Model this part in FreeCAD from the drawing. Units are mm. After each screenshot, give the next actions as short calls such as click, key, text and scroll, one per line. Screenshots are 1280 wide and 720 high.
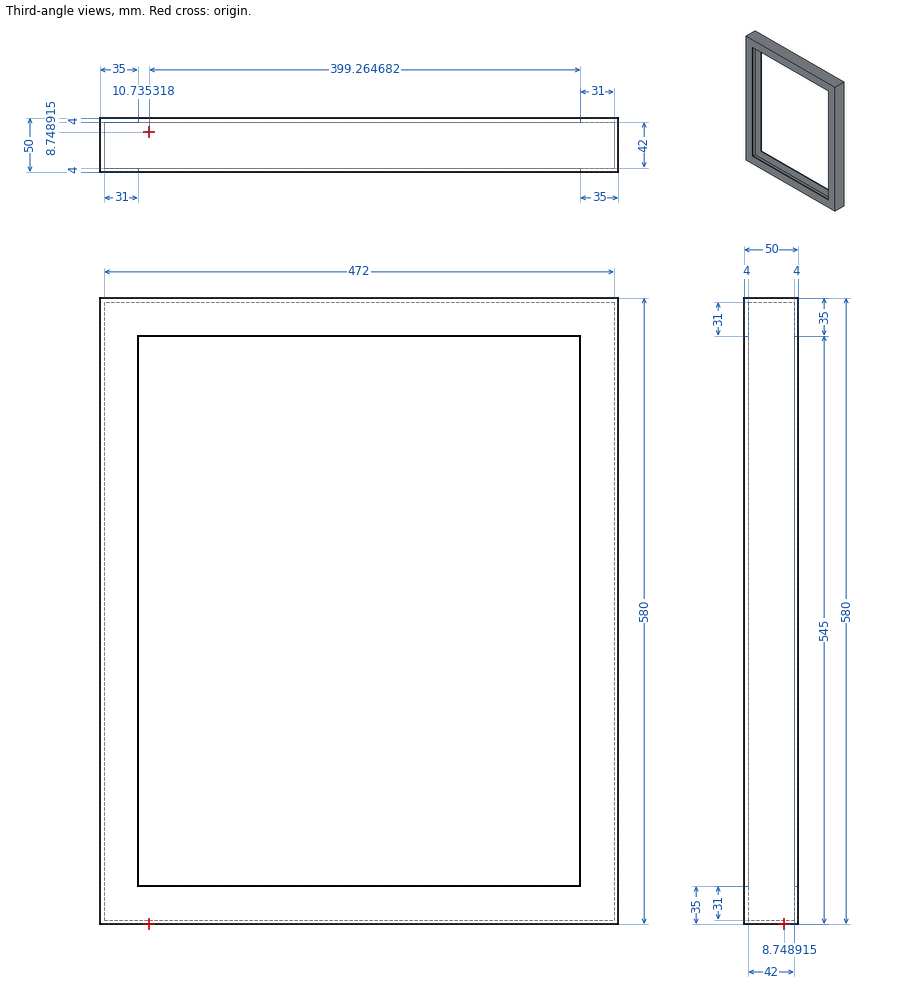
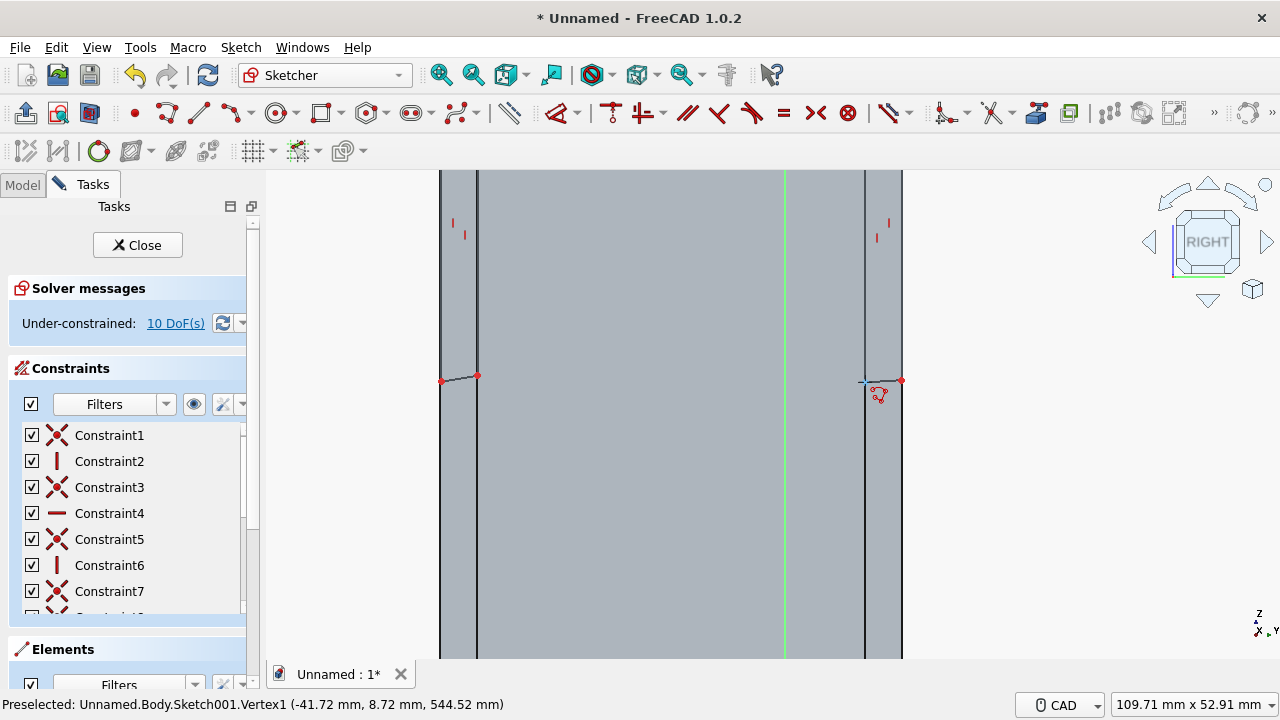
scroll(707, 264, down, 14)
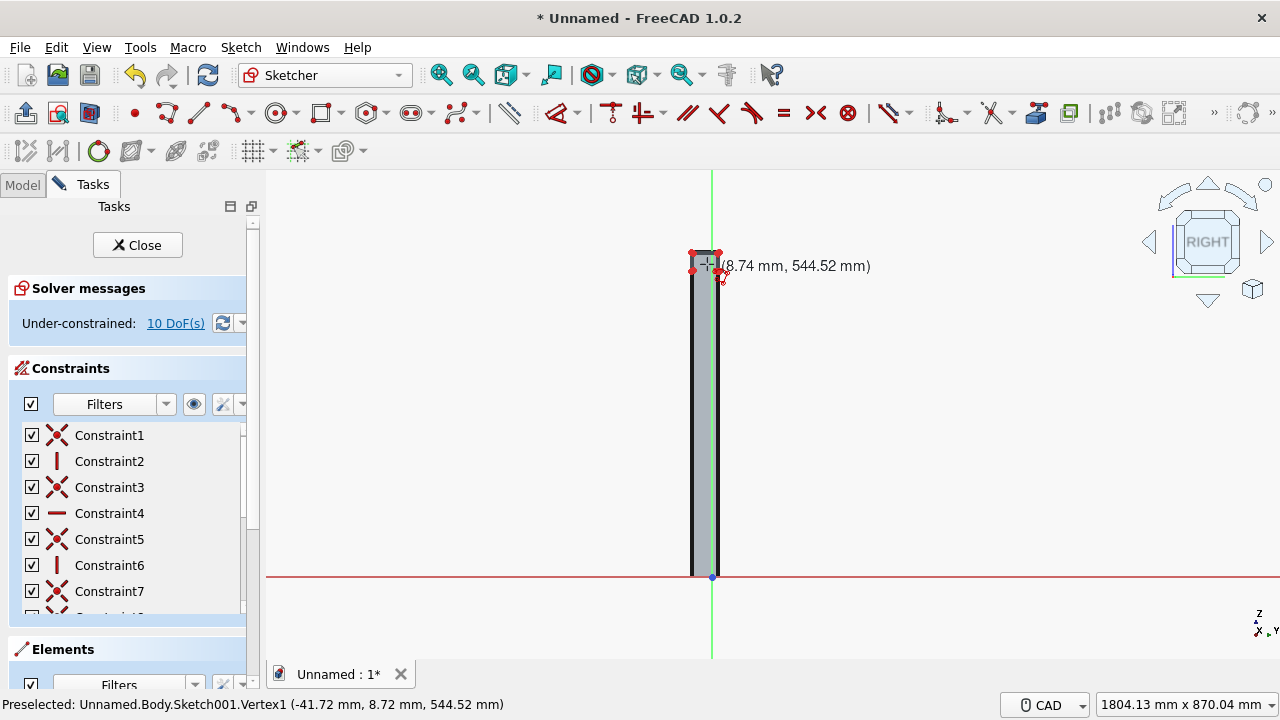
scroll(717, 575, up, 10)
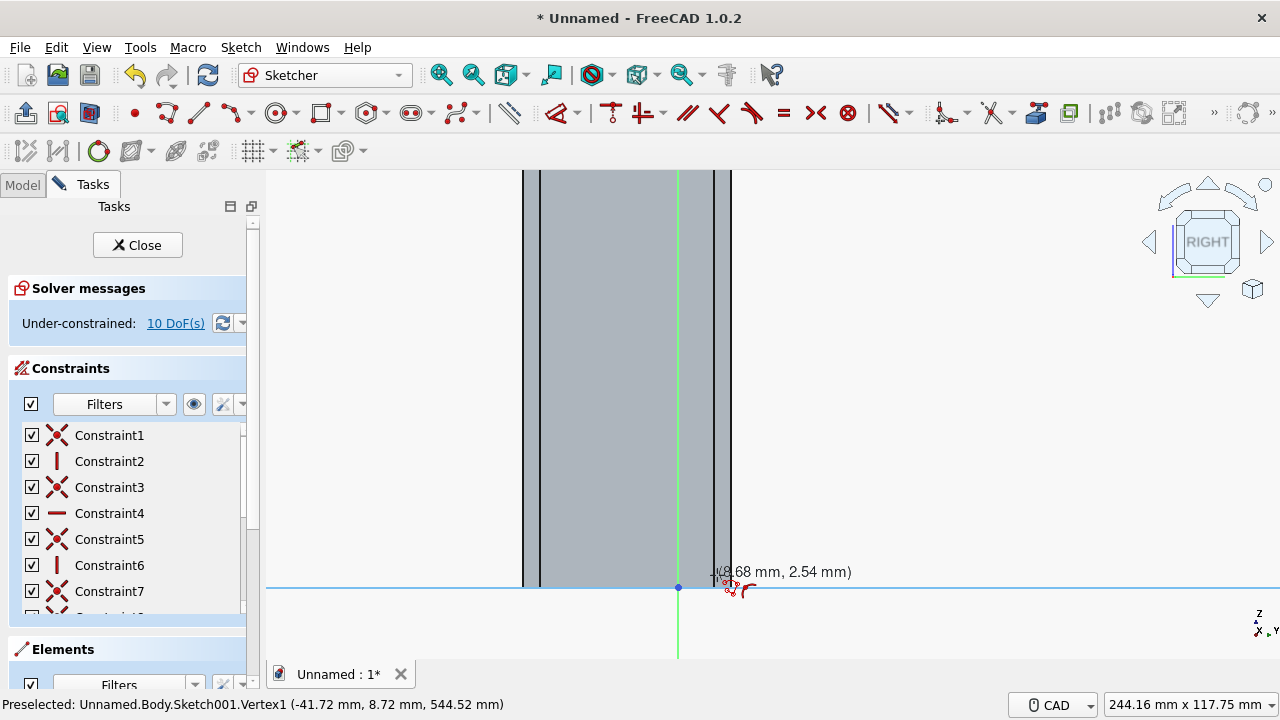
click(714, 571)
click(540, 571)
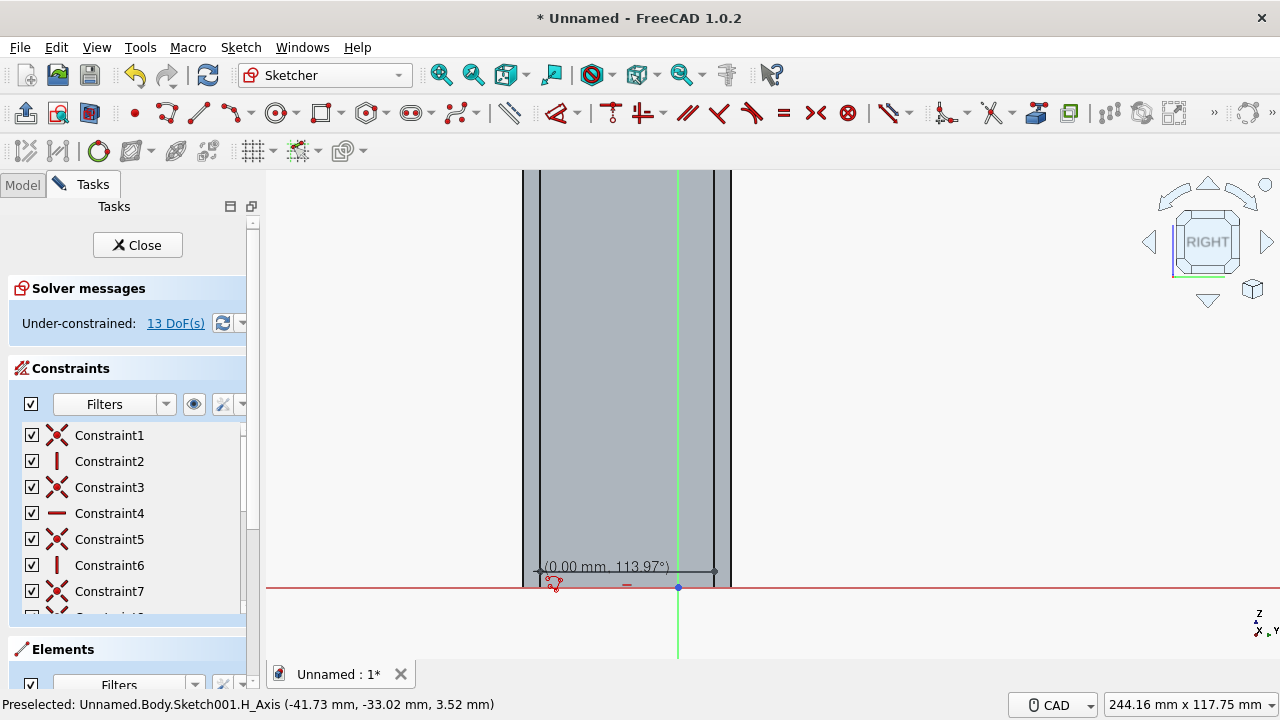
scroll(717, 576, down, 10)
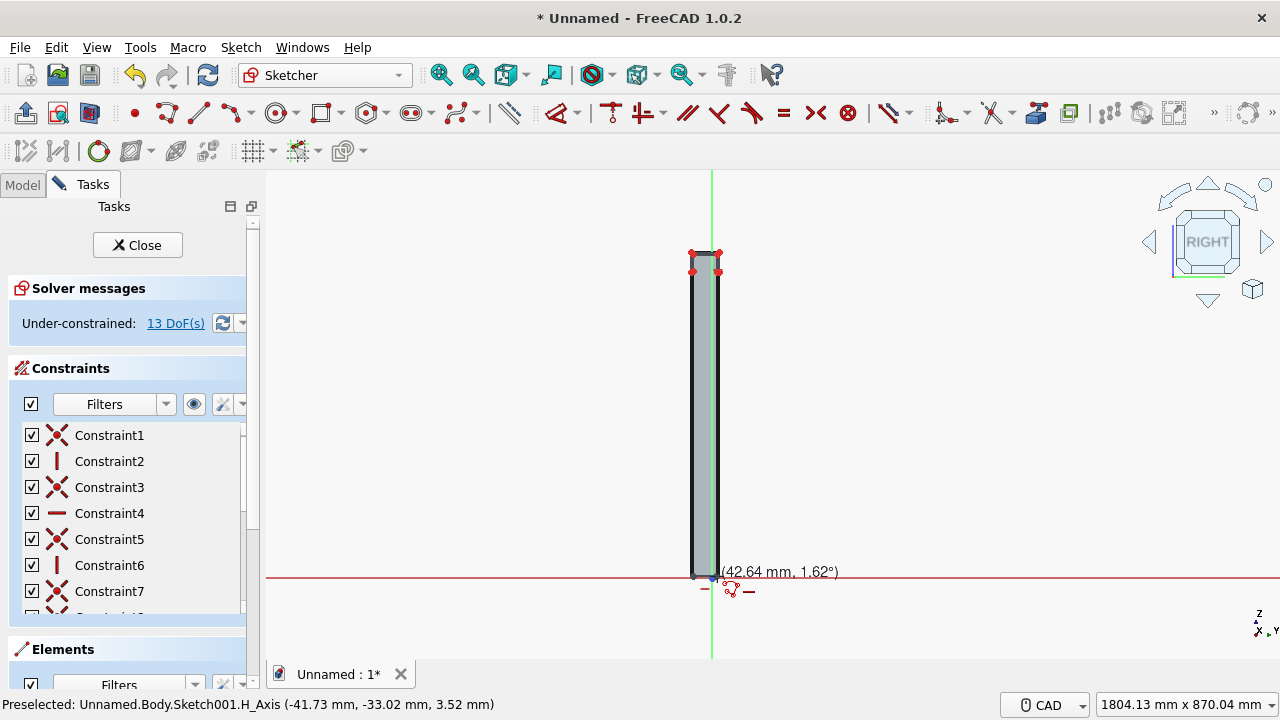
click(693, 559)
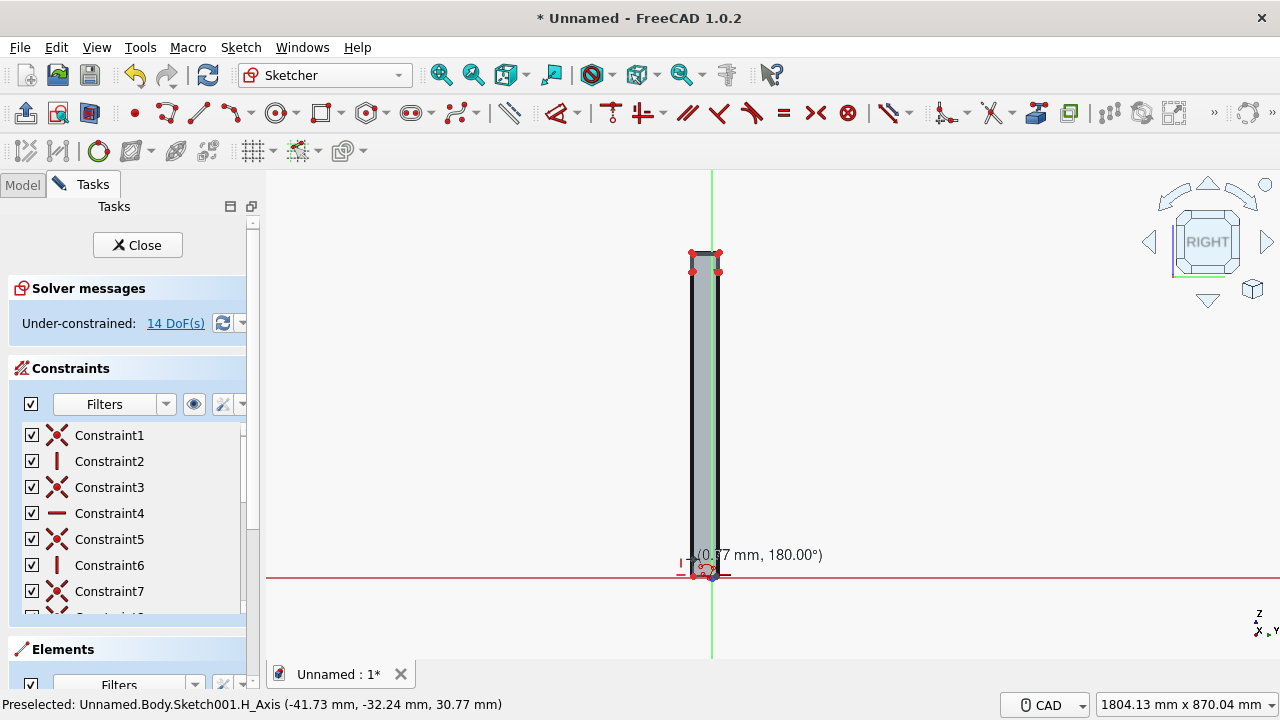
scroll(691, 559, up, 10)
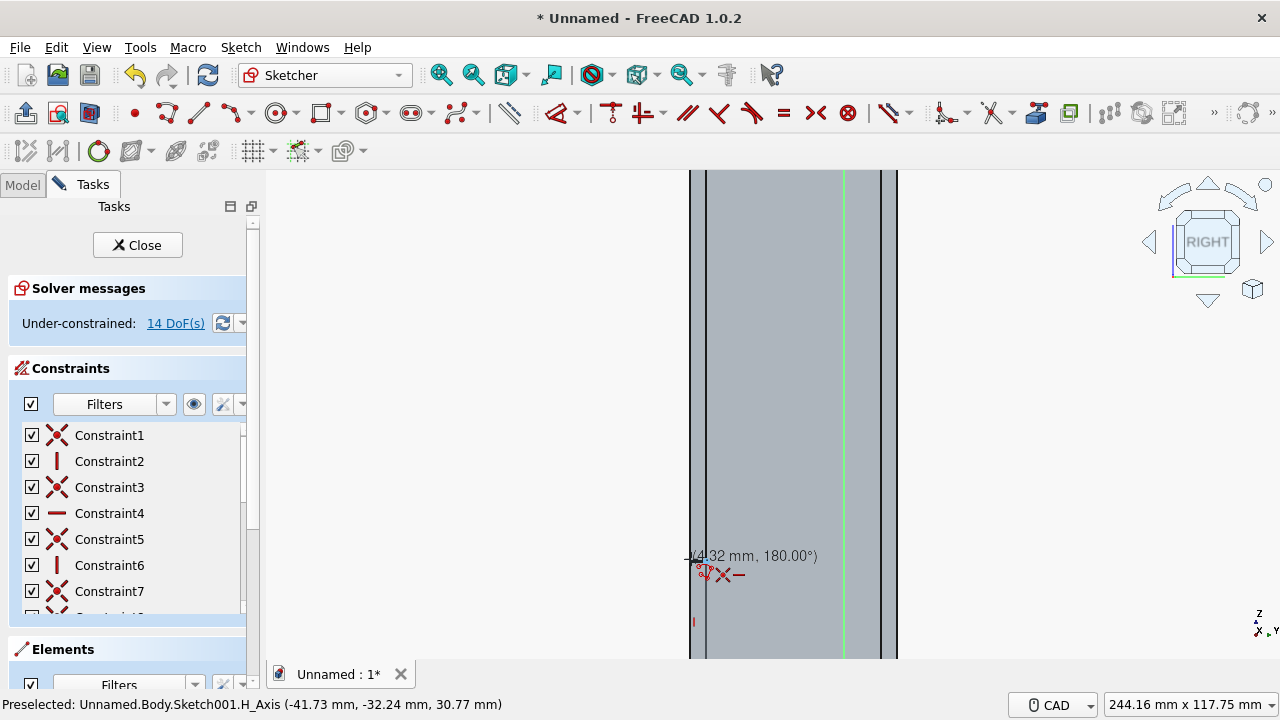
click(690, 554)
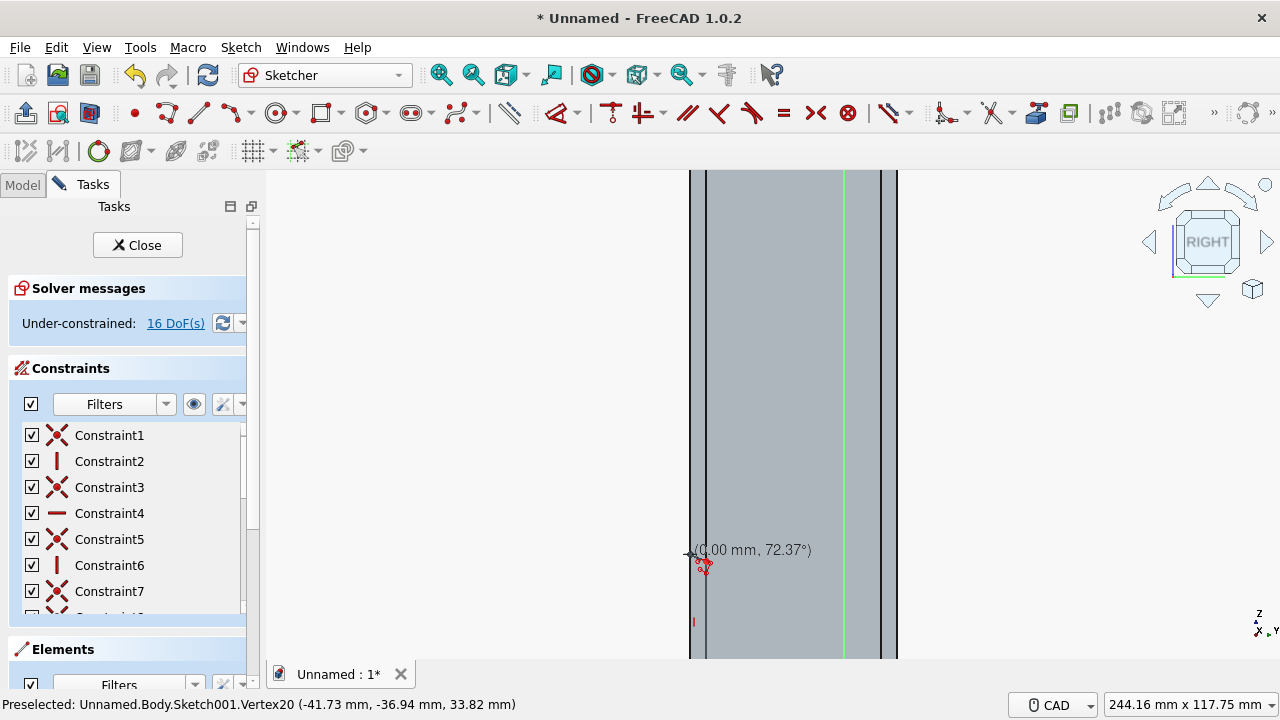
scroll(691, 559, down, 10)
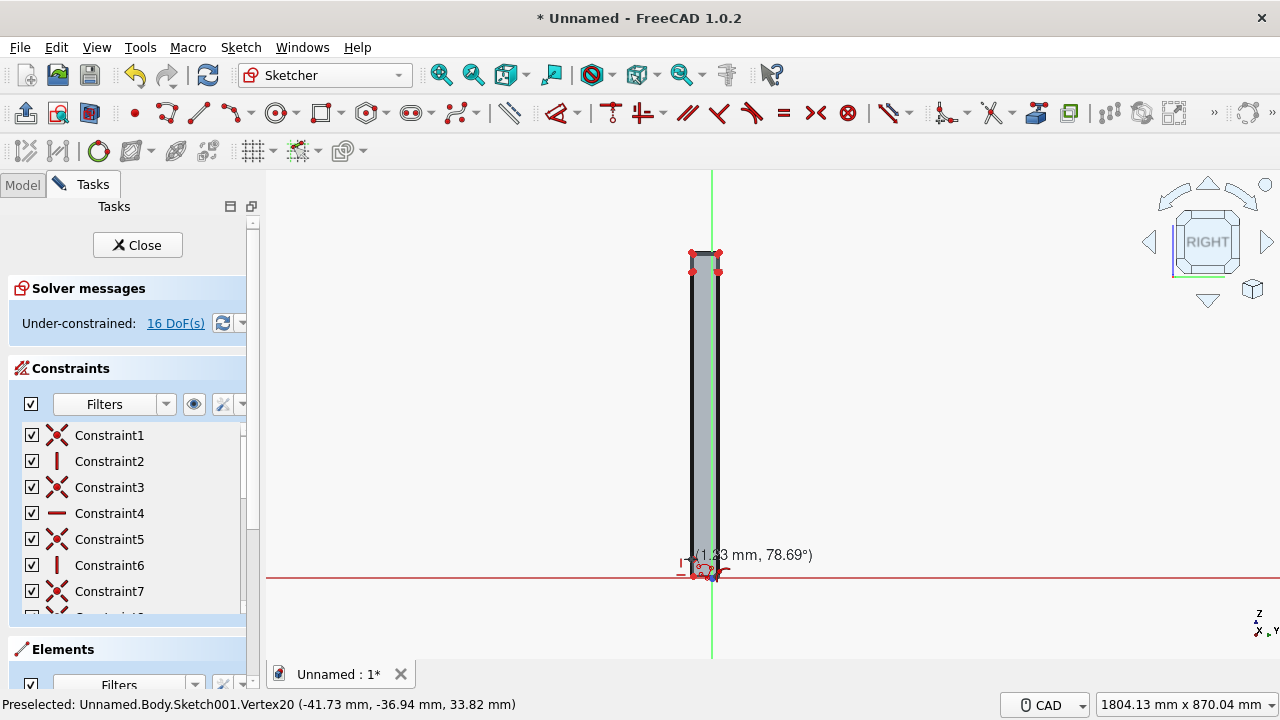
scroll(691, 578, up, 9)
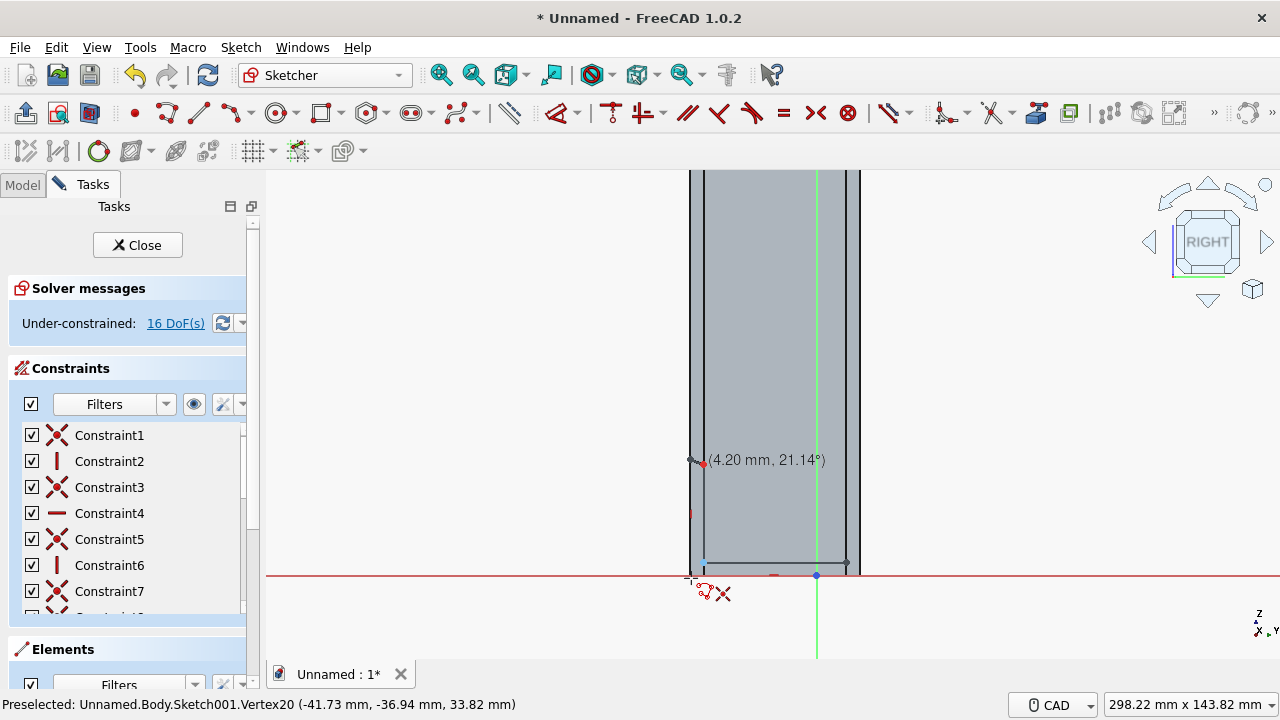
click(690, 576)
click(860, 567)
click(860, 457)
click(846, 457)
click(846, 563)
key(Escape)
key(Escape)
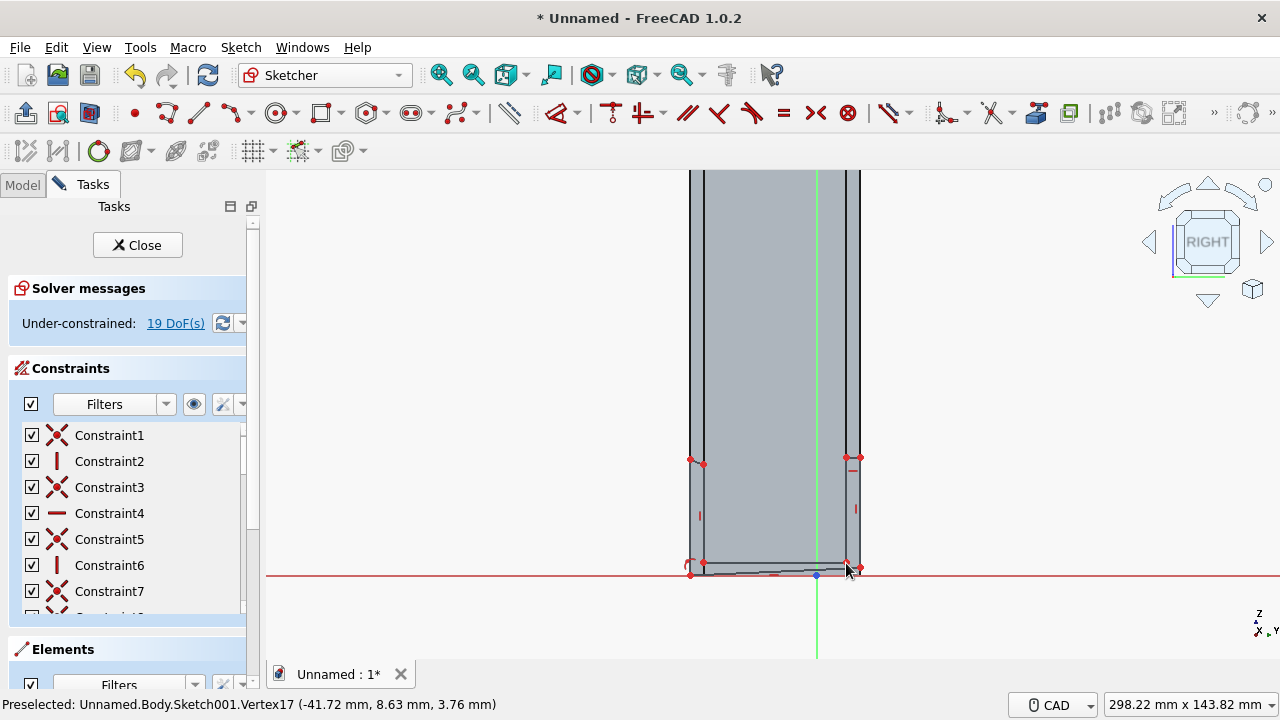
scroll(691, 578, down, 9)